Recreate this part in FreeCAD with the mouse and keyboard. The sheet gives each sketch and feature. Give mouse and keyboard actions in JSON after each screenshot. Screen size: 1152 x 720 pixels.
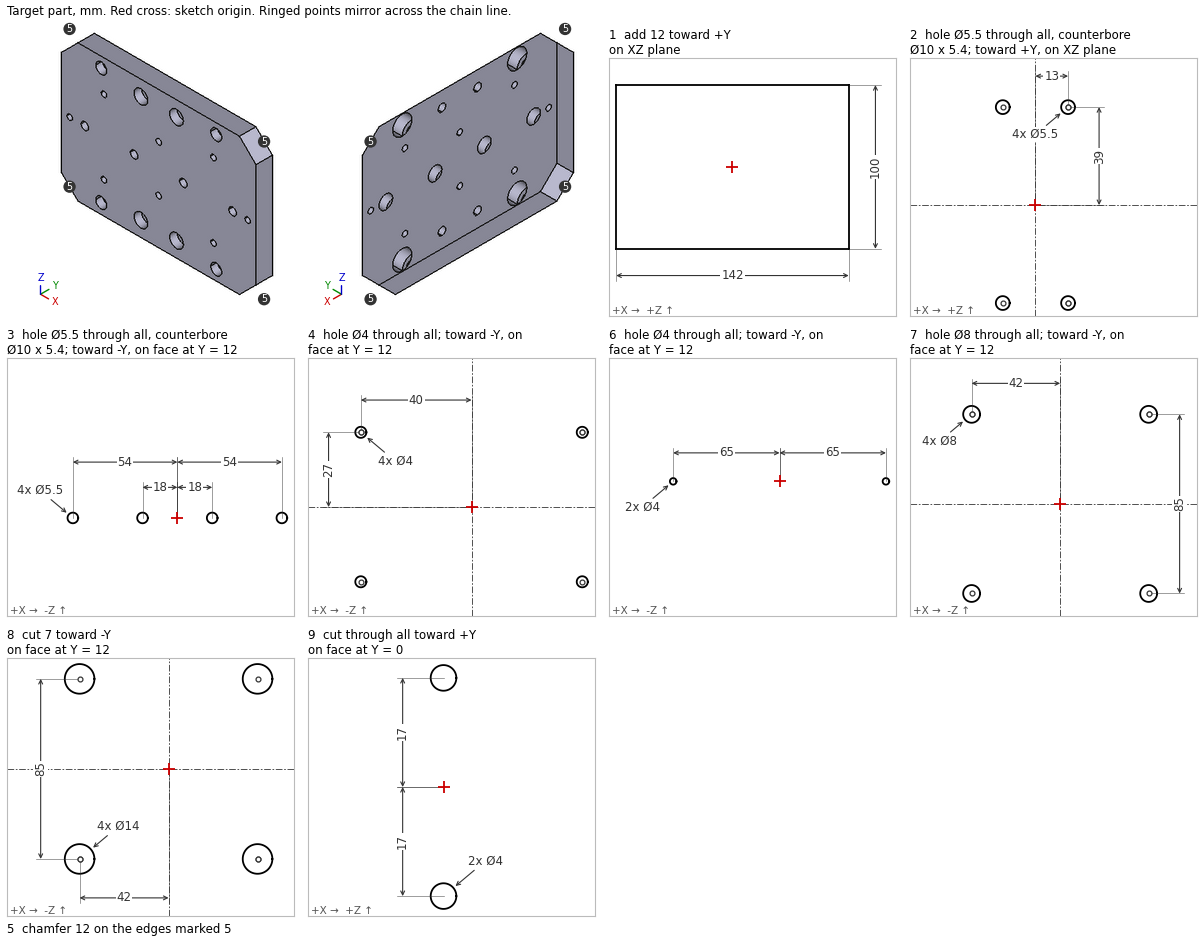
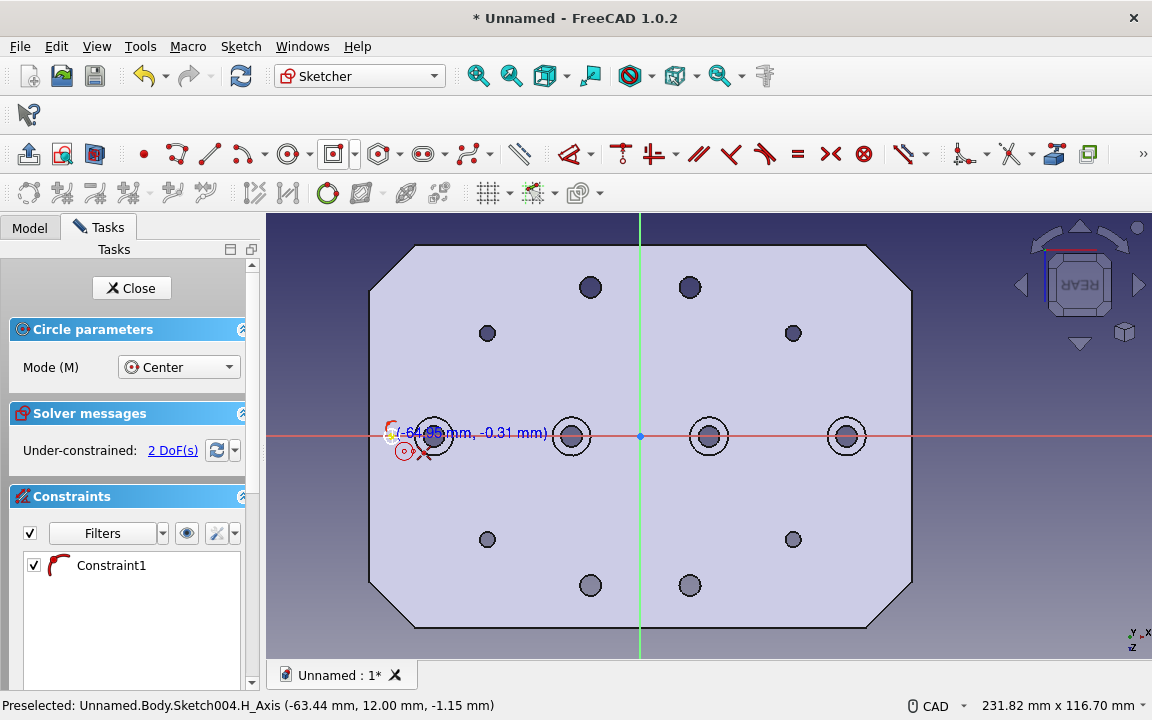
{"action": "scroll", "coordinate": [889, 436], "scroll_direction": "up", "scroll_amount": 6}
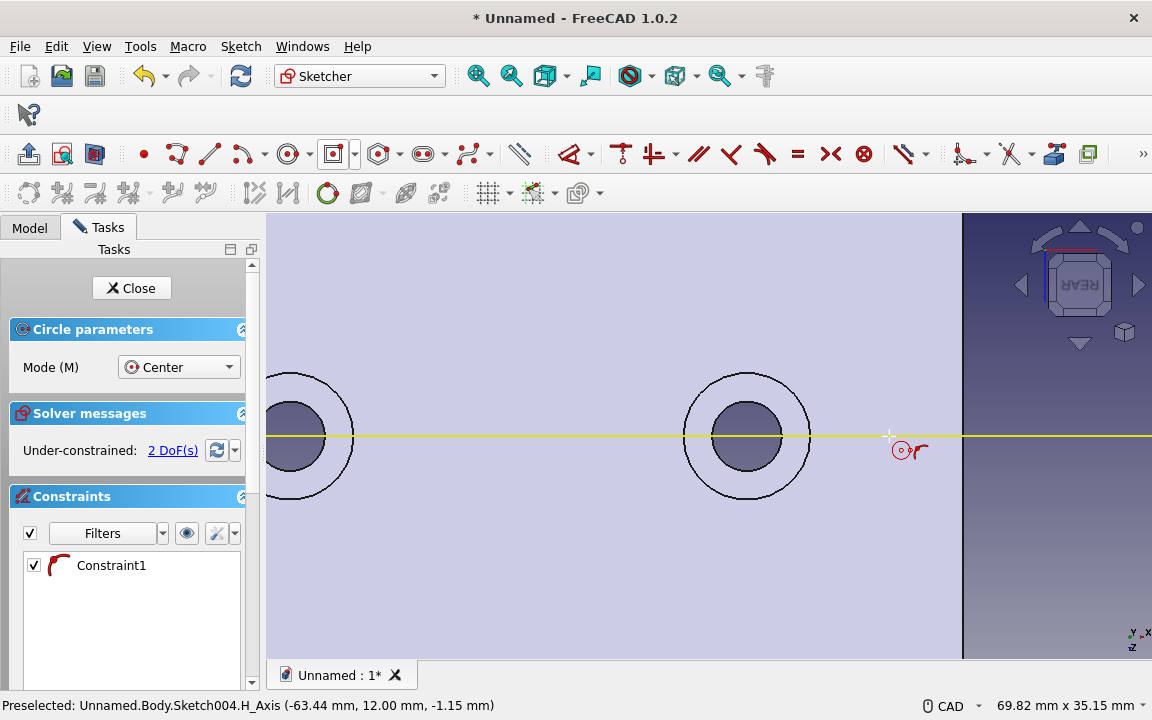
{"action": "left_click", "coordinate": [886, 436]}
{"action": "left_click", "coordinate": [904, 418]}
{"action": "key", "text": "Escape"}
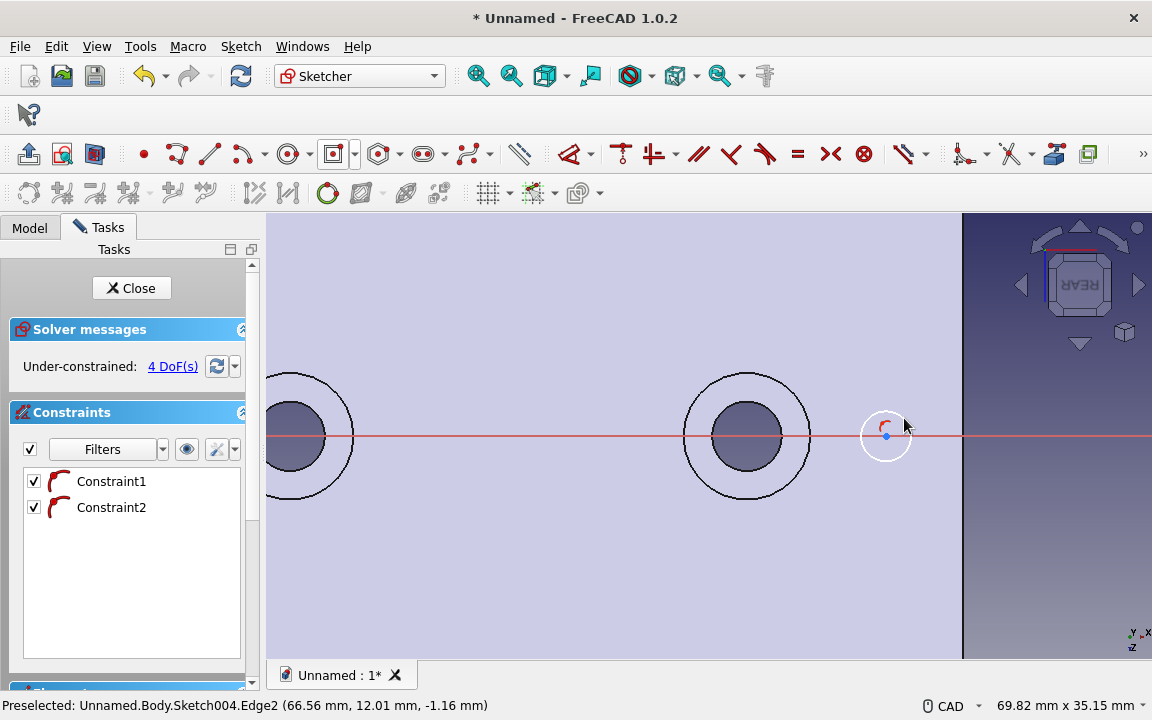
{"action": "scroll", "coordinate": [890, 436], "scroll_direction": "down", "scroll_amount": 6}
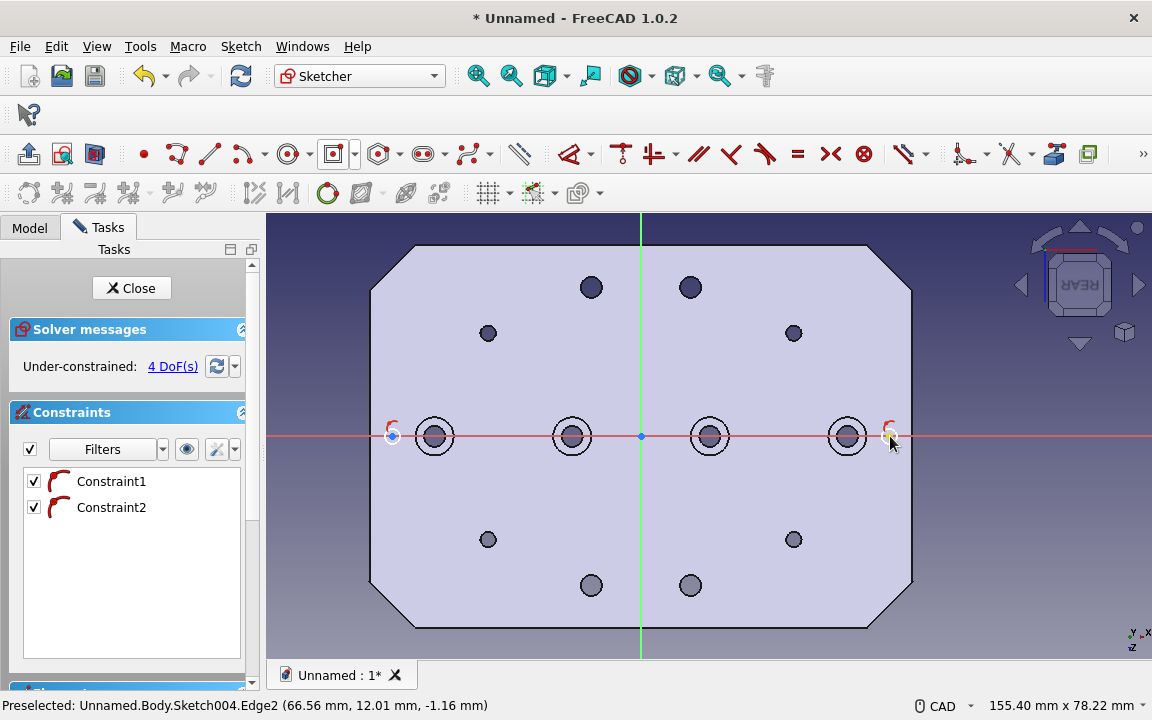
{"action": "scroll", "coordinate": [398, 431], "scroll_direction": "up", "scroll_amount": 5}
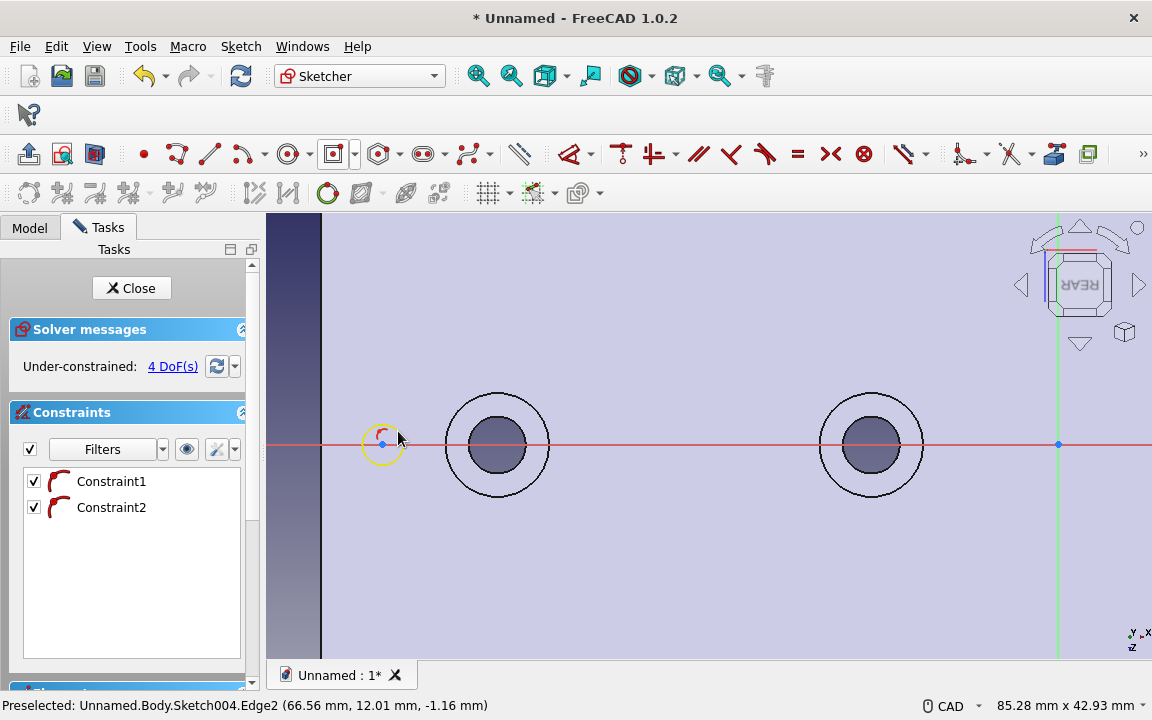
{"action": "left_click", "coordinate": [397, 431]}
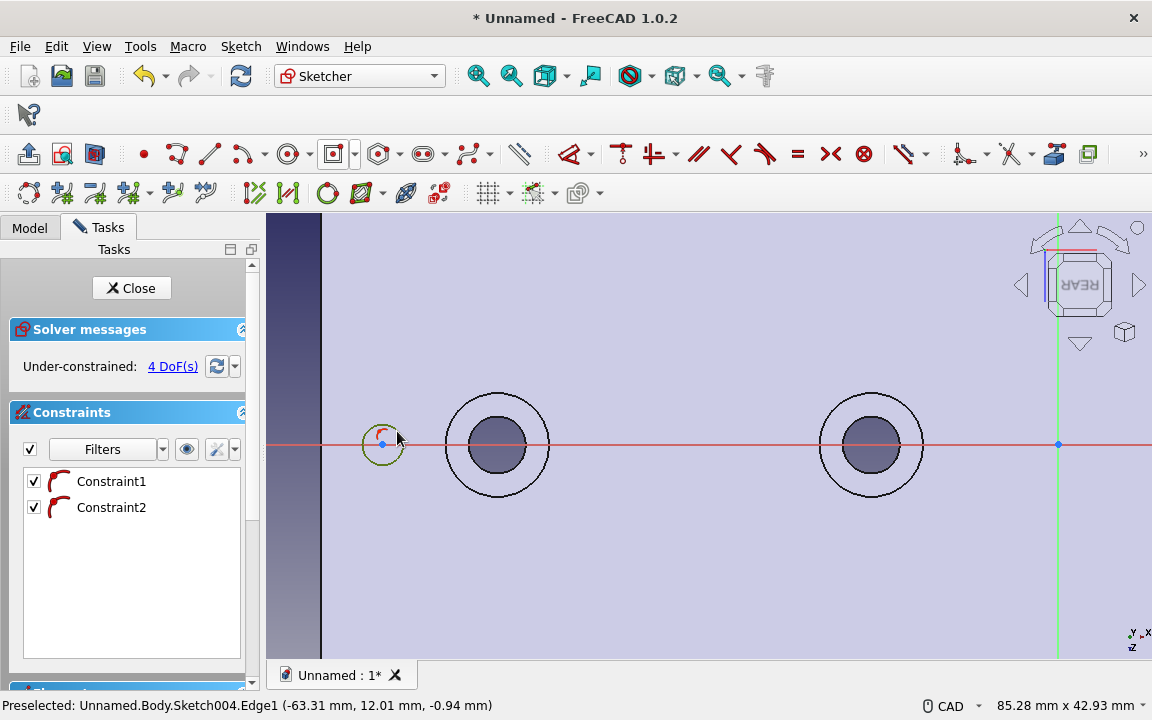
{"action": "scroll", "coordinate": [397, 431], "scroll_direction": "down", "scroll_amount": 5}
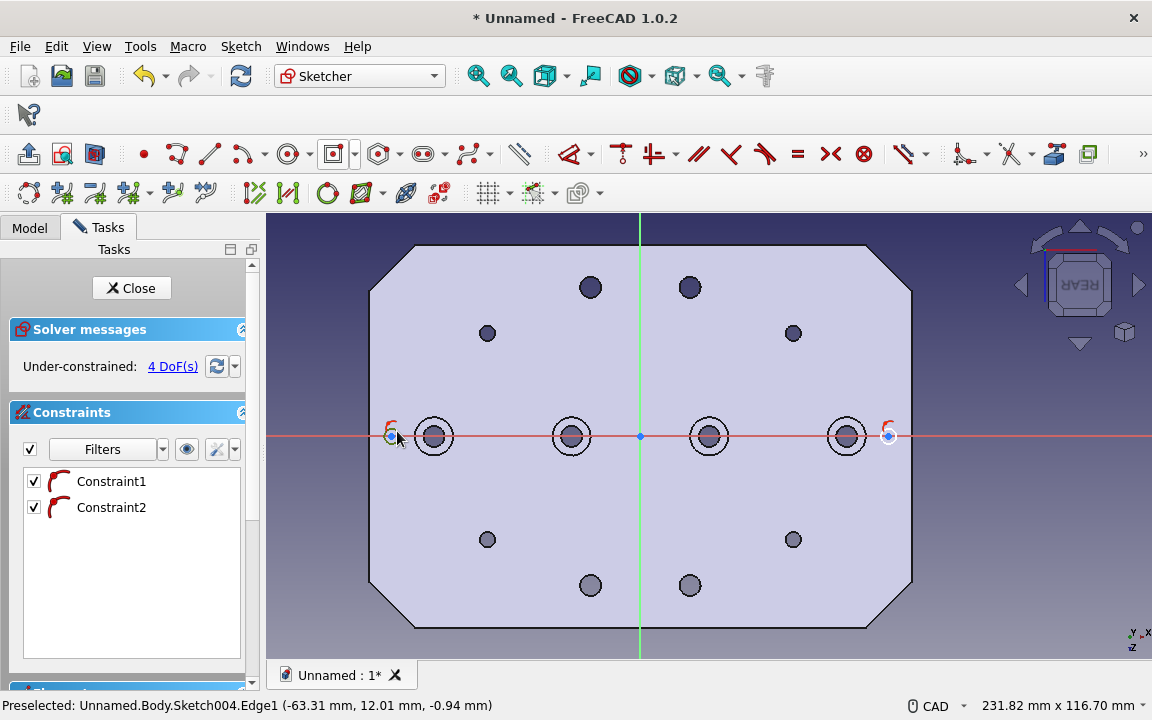
{"action": "scroll", "coordinate": [894, 431], "scroll_direction": "up", "scroll_amount": 5}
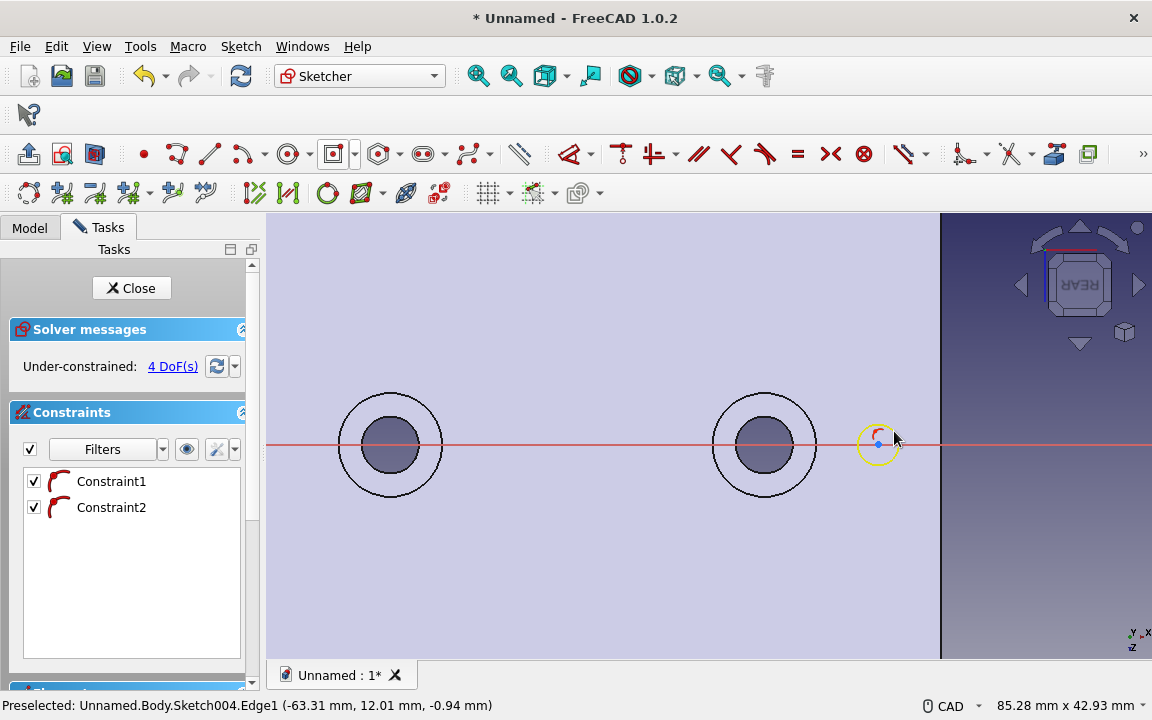
{"action": "left_click", "coordinate": [893, 430]}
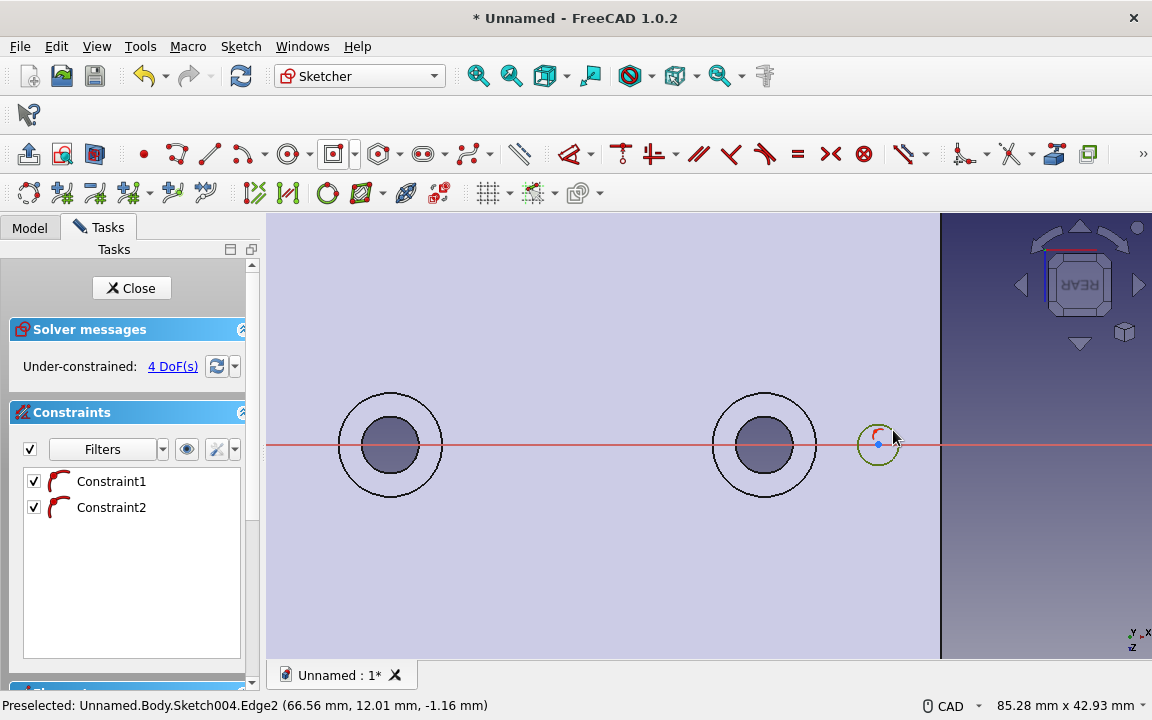
{"action": "left_click", "coordinate": [798, 154]}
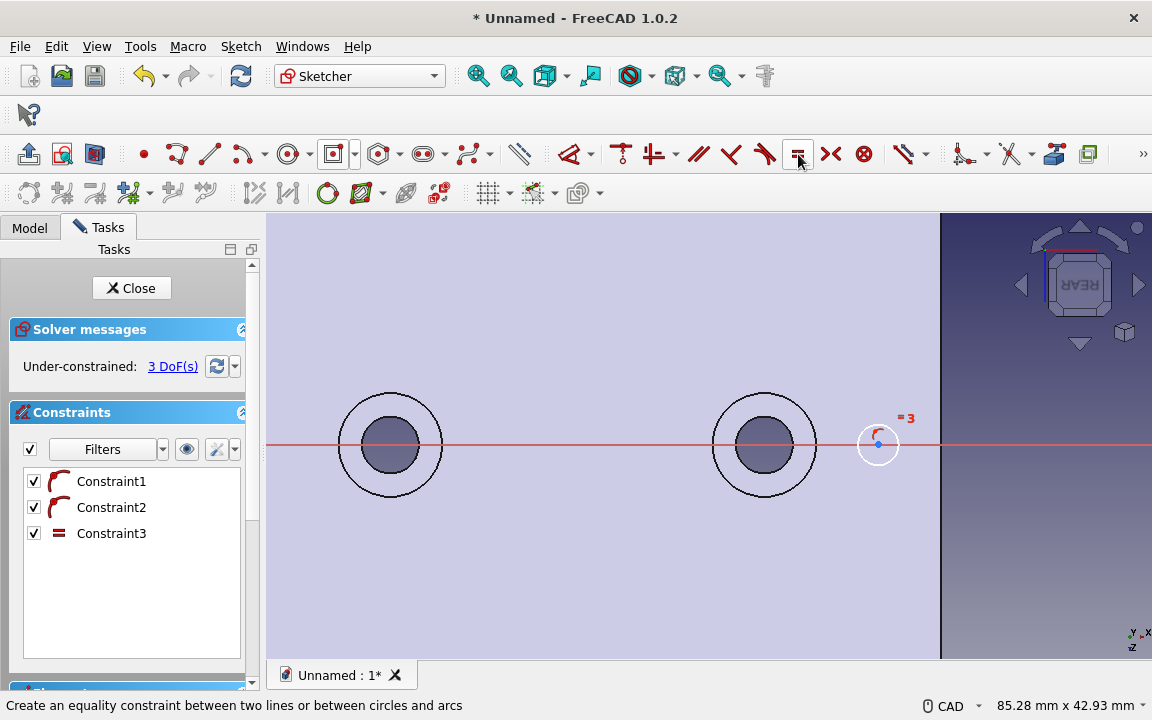
{"action": "left_click", "coordinate": [568, 154]}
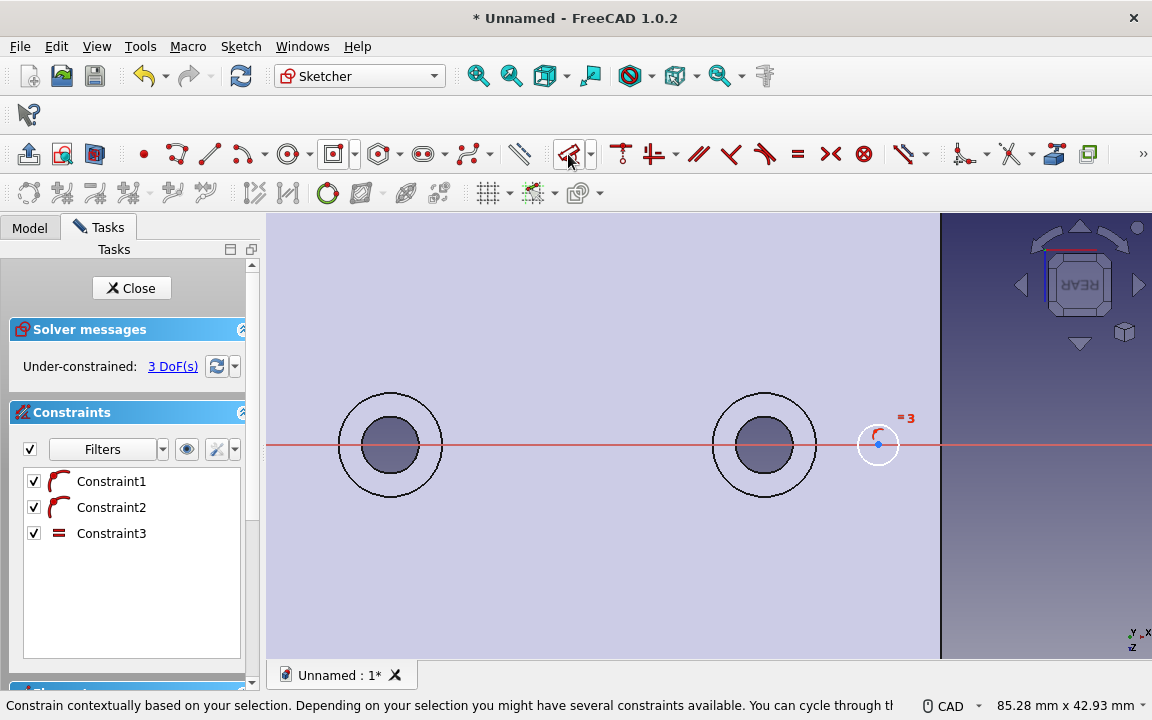
{"action": "scroll", "coordinate": [895, 431], "scroll_direction": "down", "scroll_amount": 5}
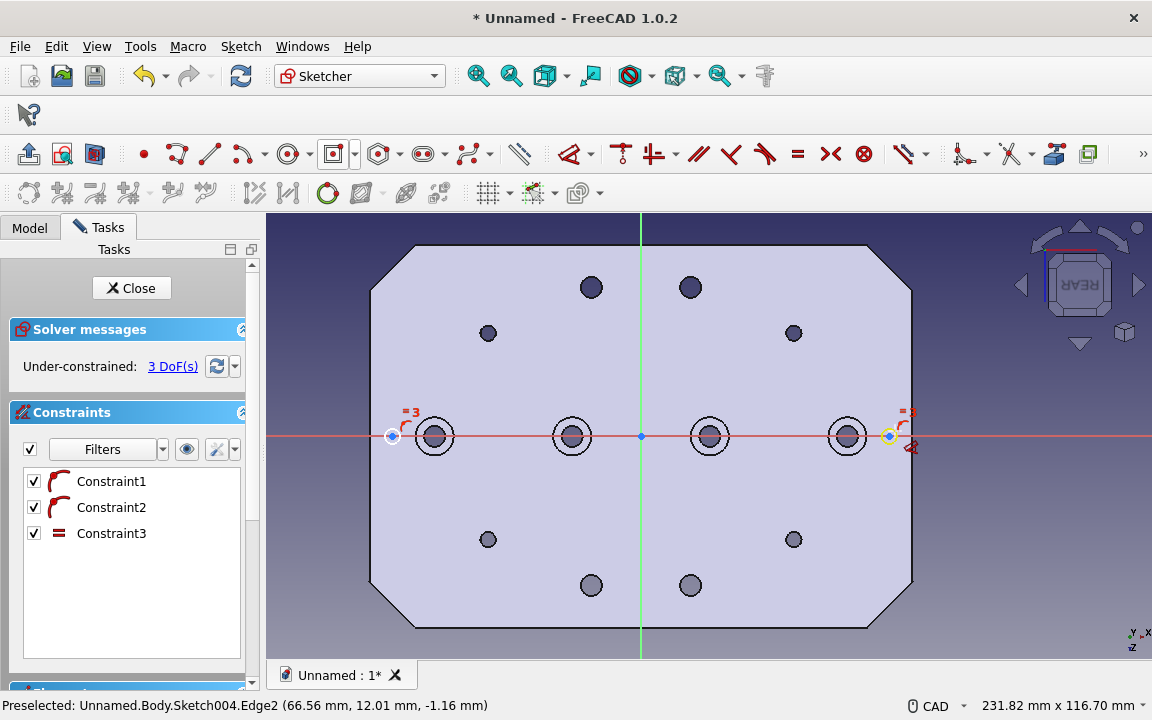
{"action": "scroll", "coordinate": [398, 431], "scroll_direction": "up", "scroll_amount": 5}